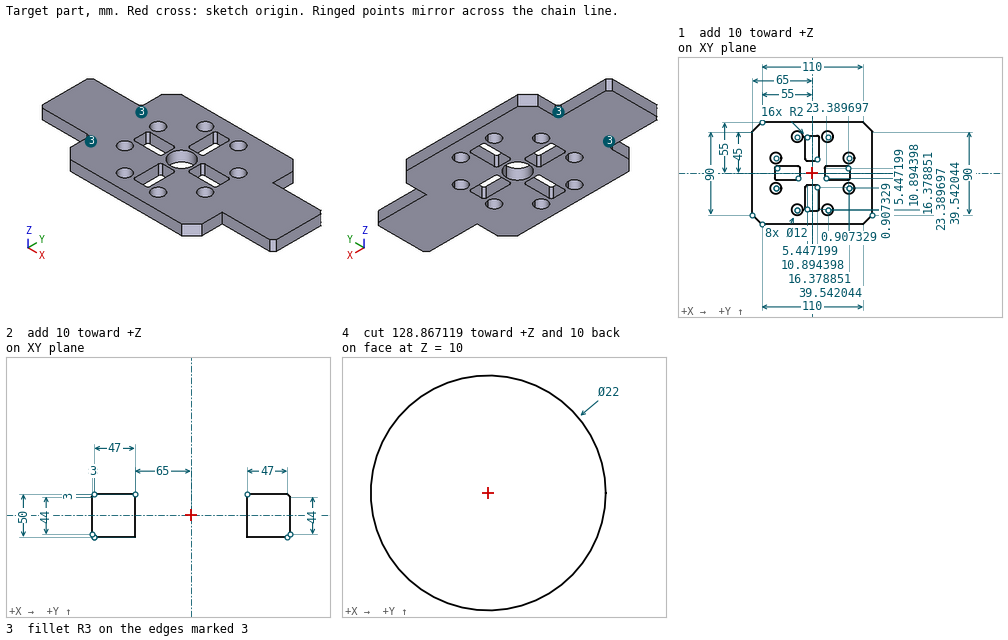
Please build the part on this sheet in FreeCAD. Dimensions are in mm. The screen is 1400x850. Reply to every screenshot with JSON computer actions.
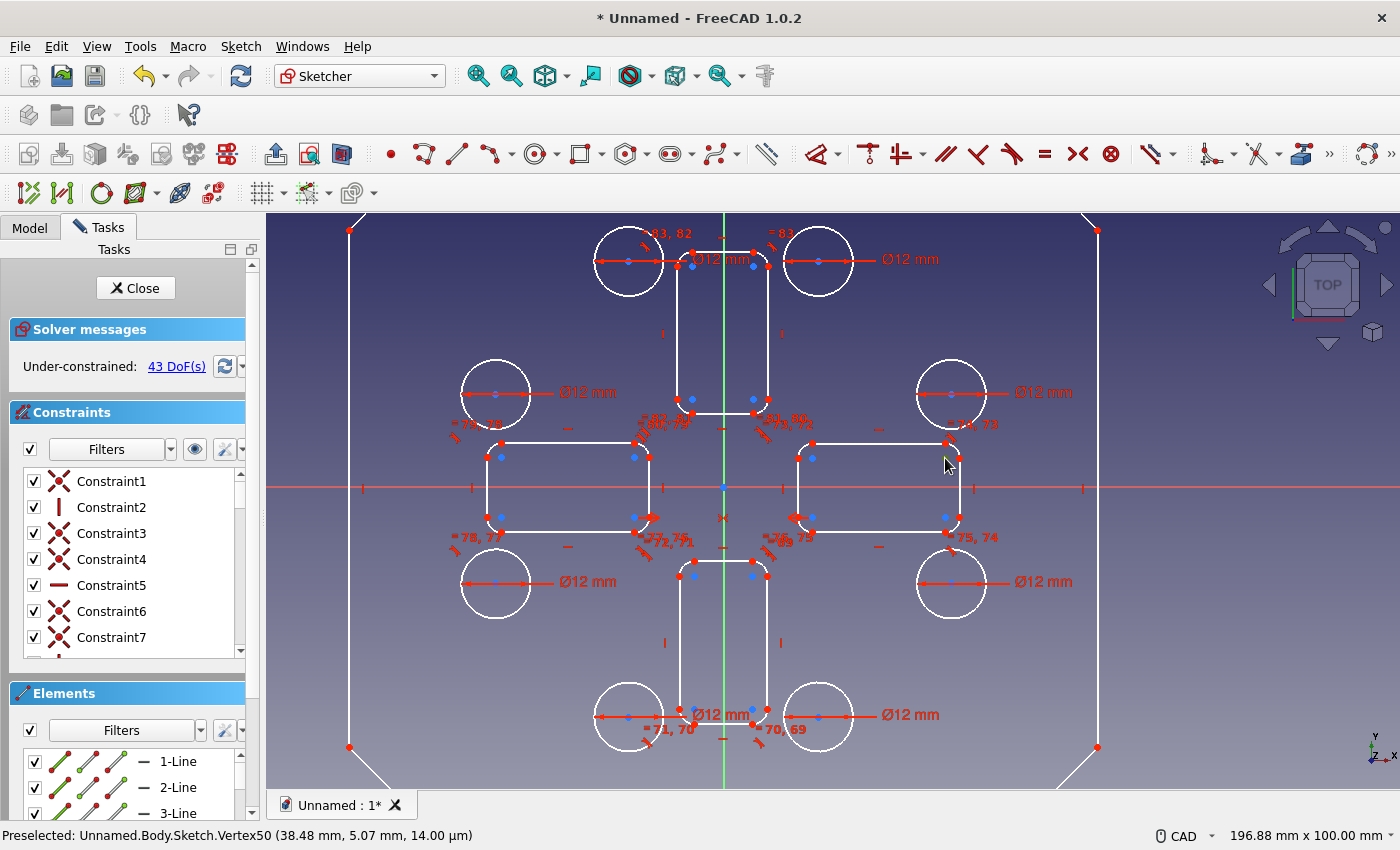
{"action": "left_click", "coordinate": [502, 458]}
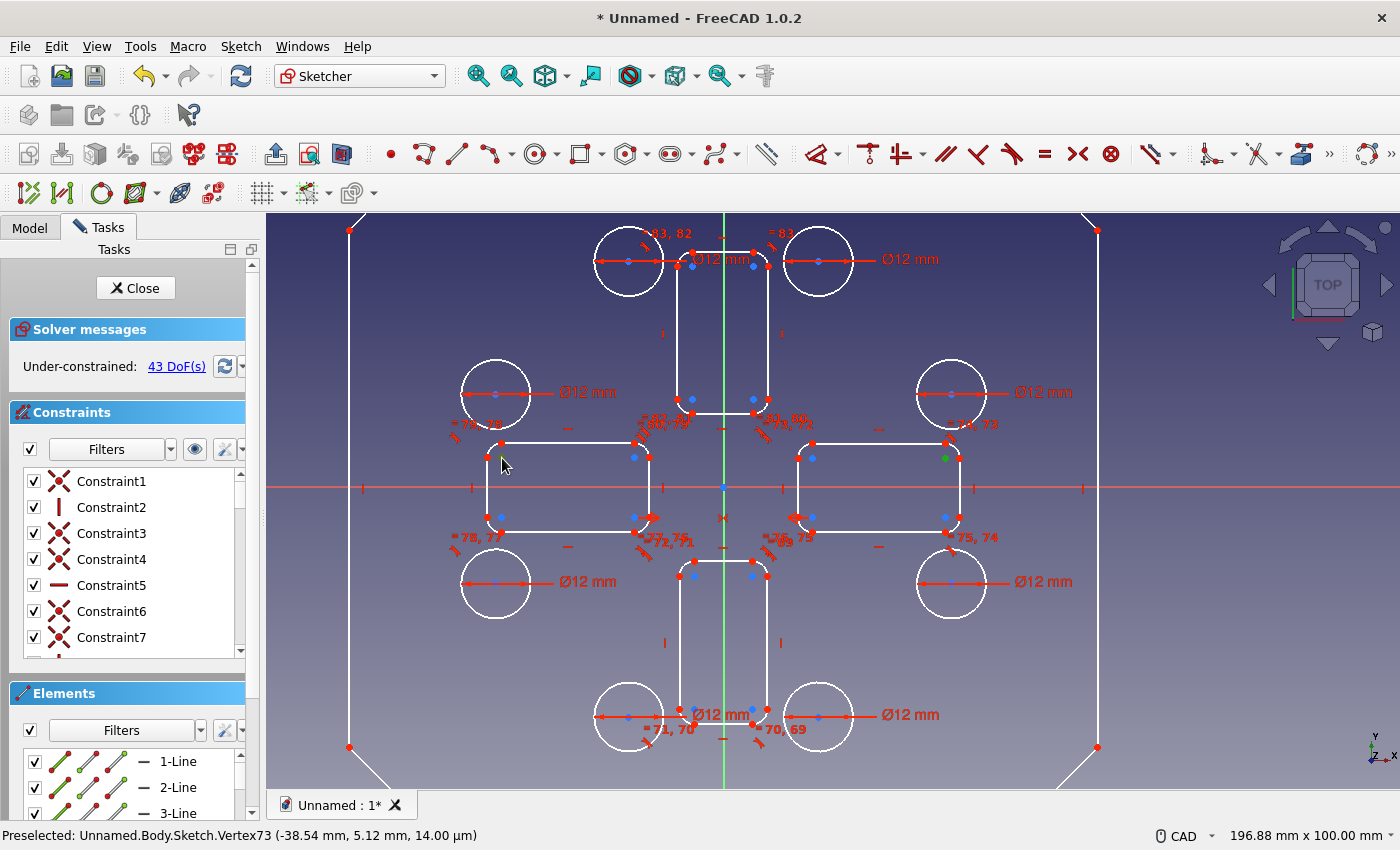
{"action": "left_click", "coordinate": [724, 687]}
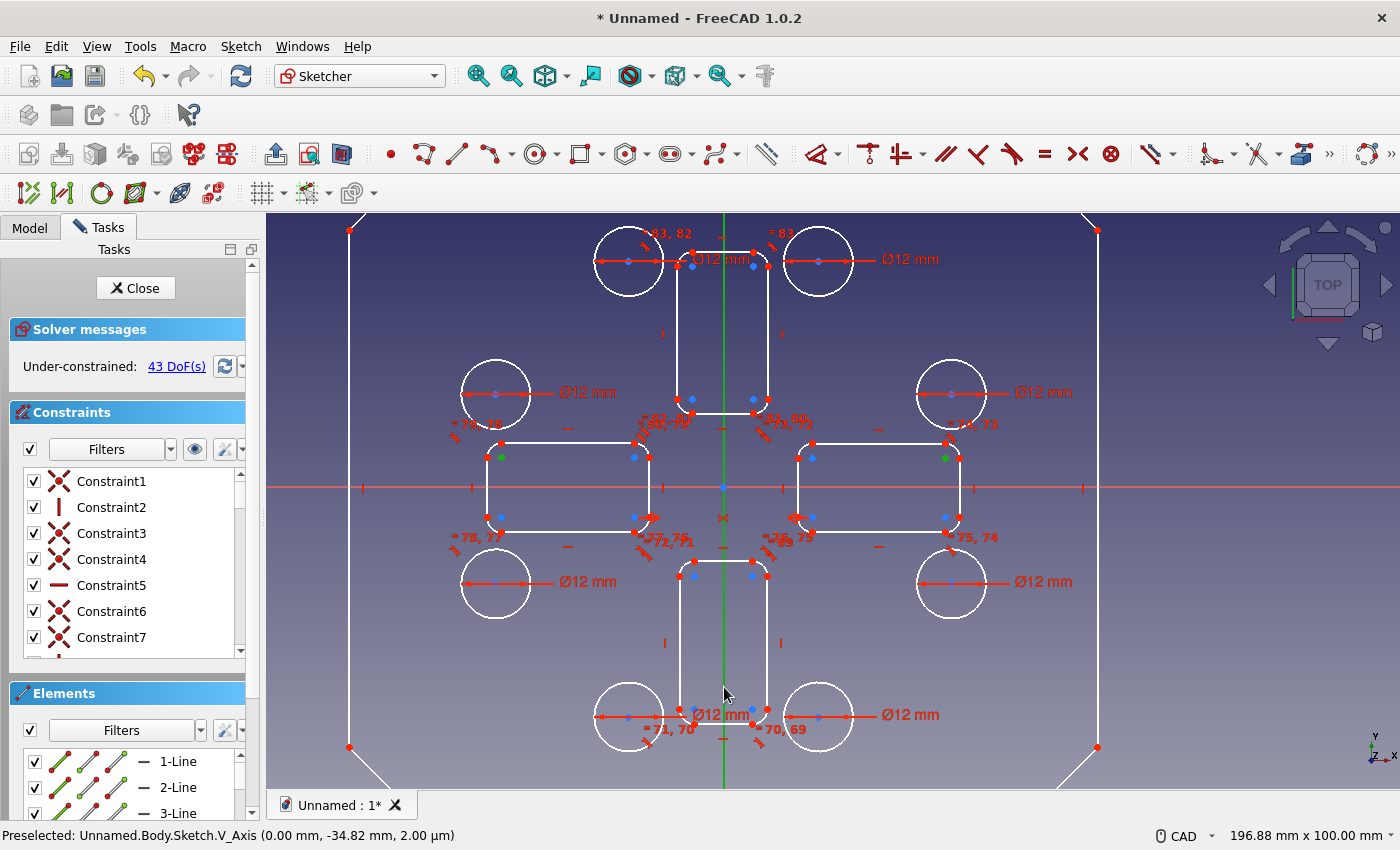
{"action": "left_click", "coordinate": [1078, 154]}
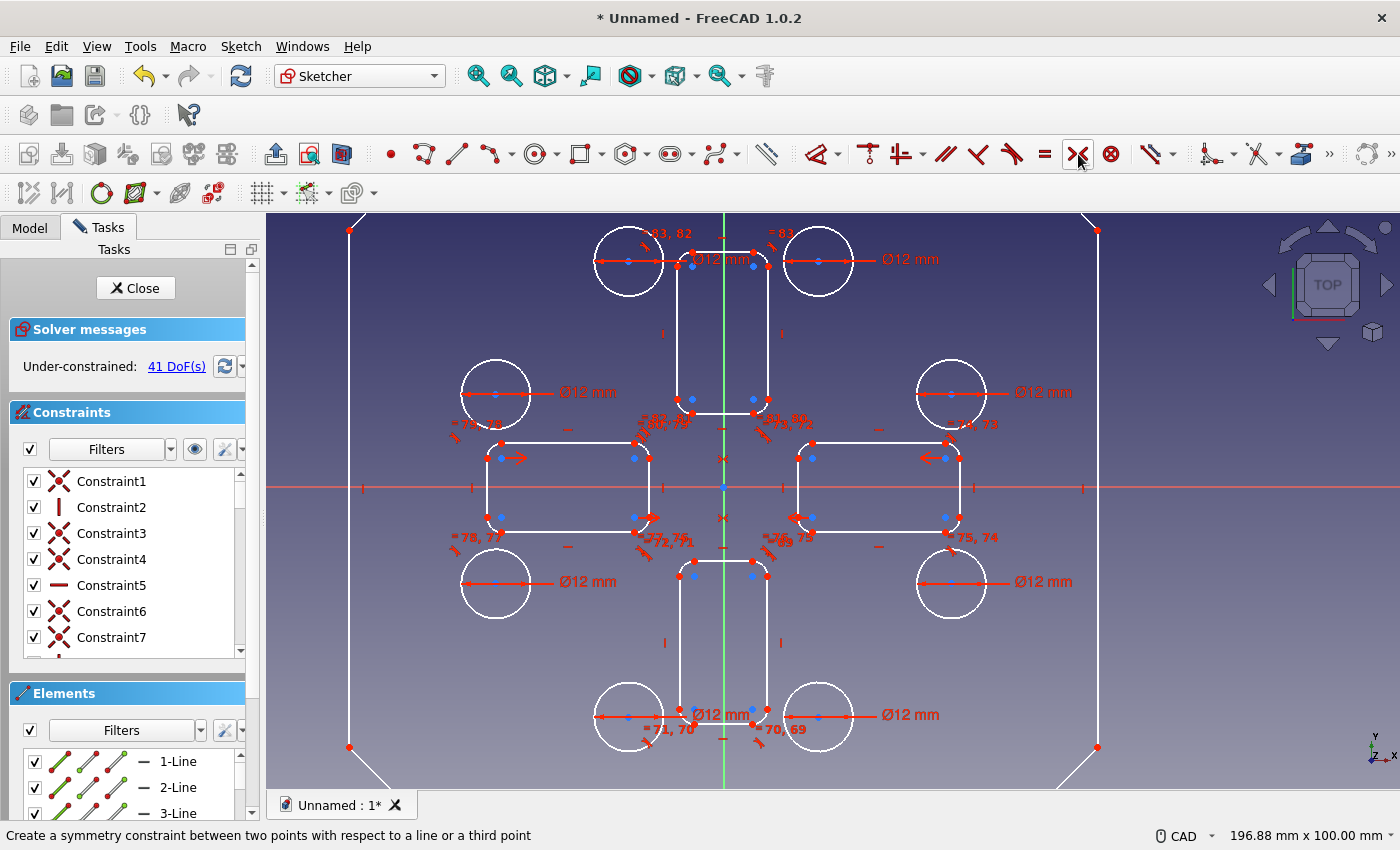
{"action": "left_click", "coordinate": [753, 576]}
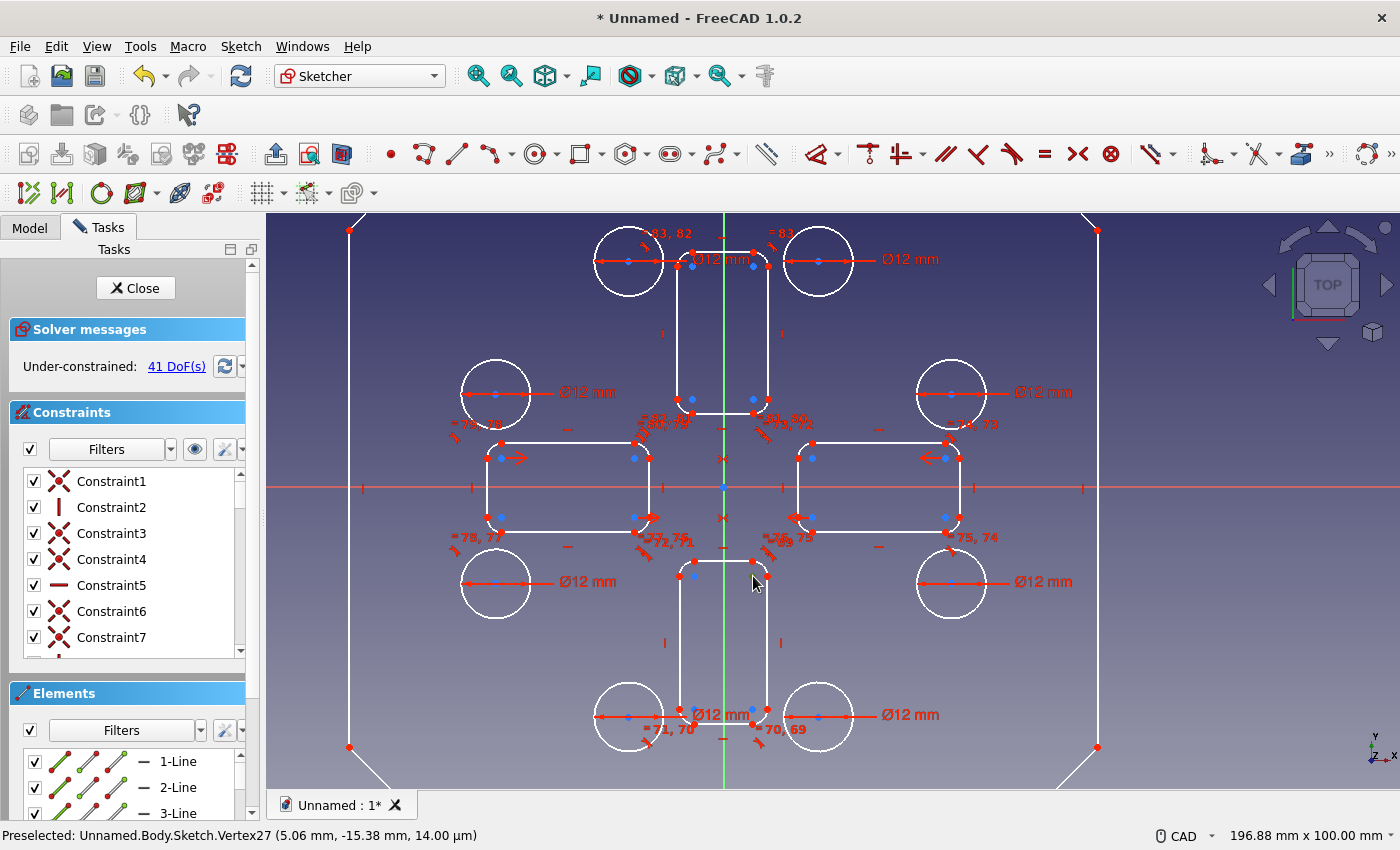
{"action": "left_click", "coordinate": [753, 399]}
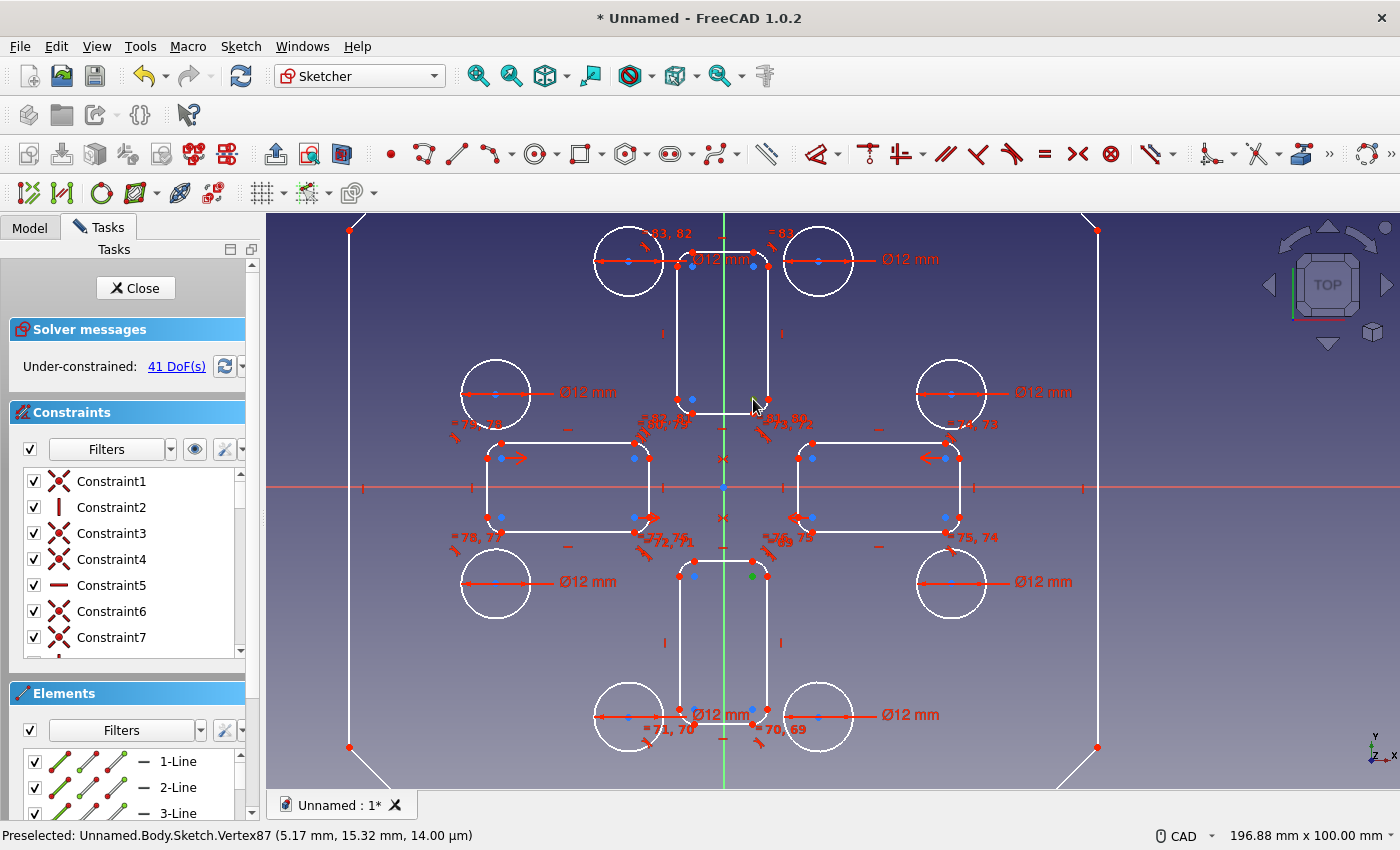
{"action": "left_click", "coordinate": [428, 487]}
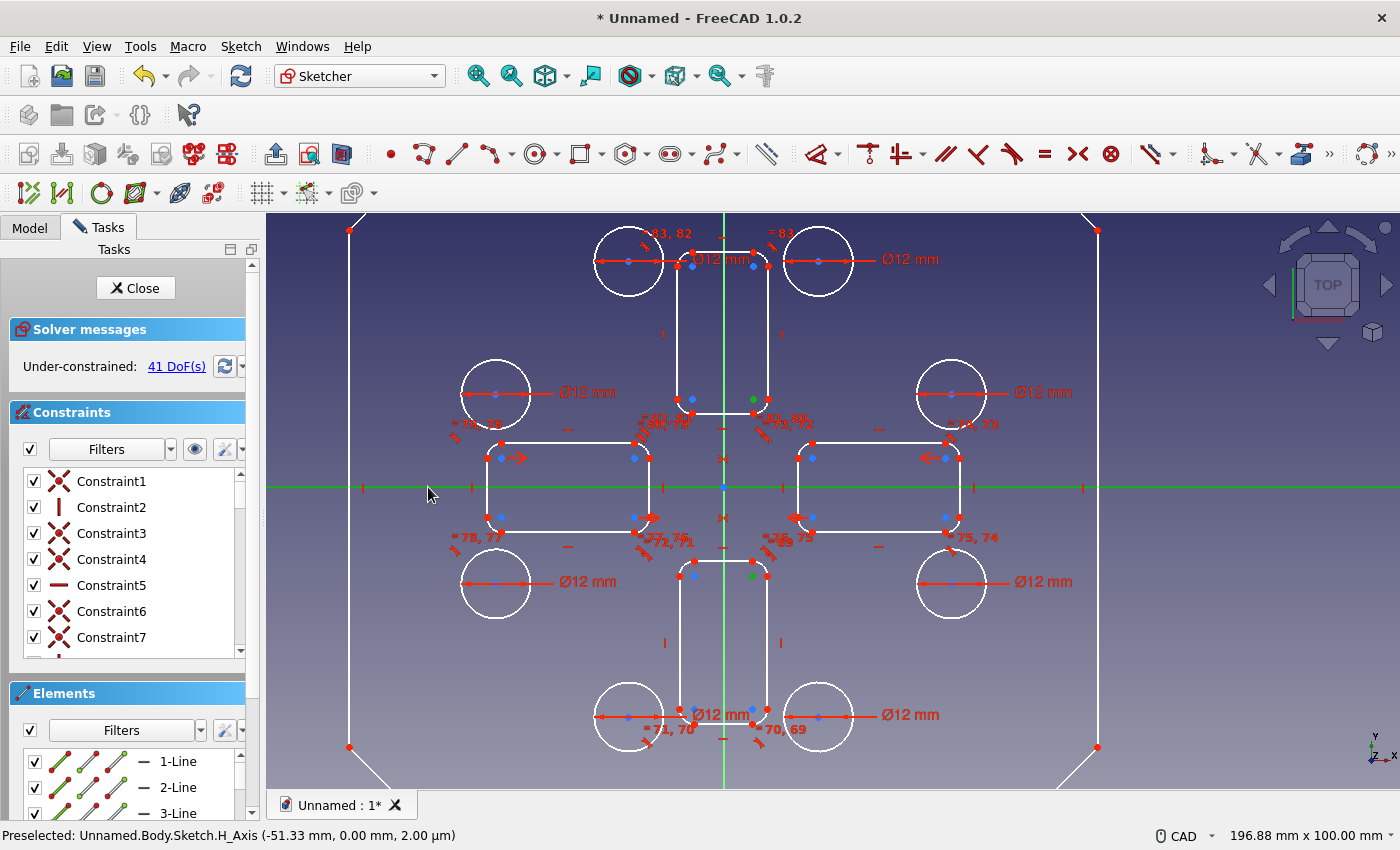
{"action": "left_click", "coordinate": [1078, 154]}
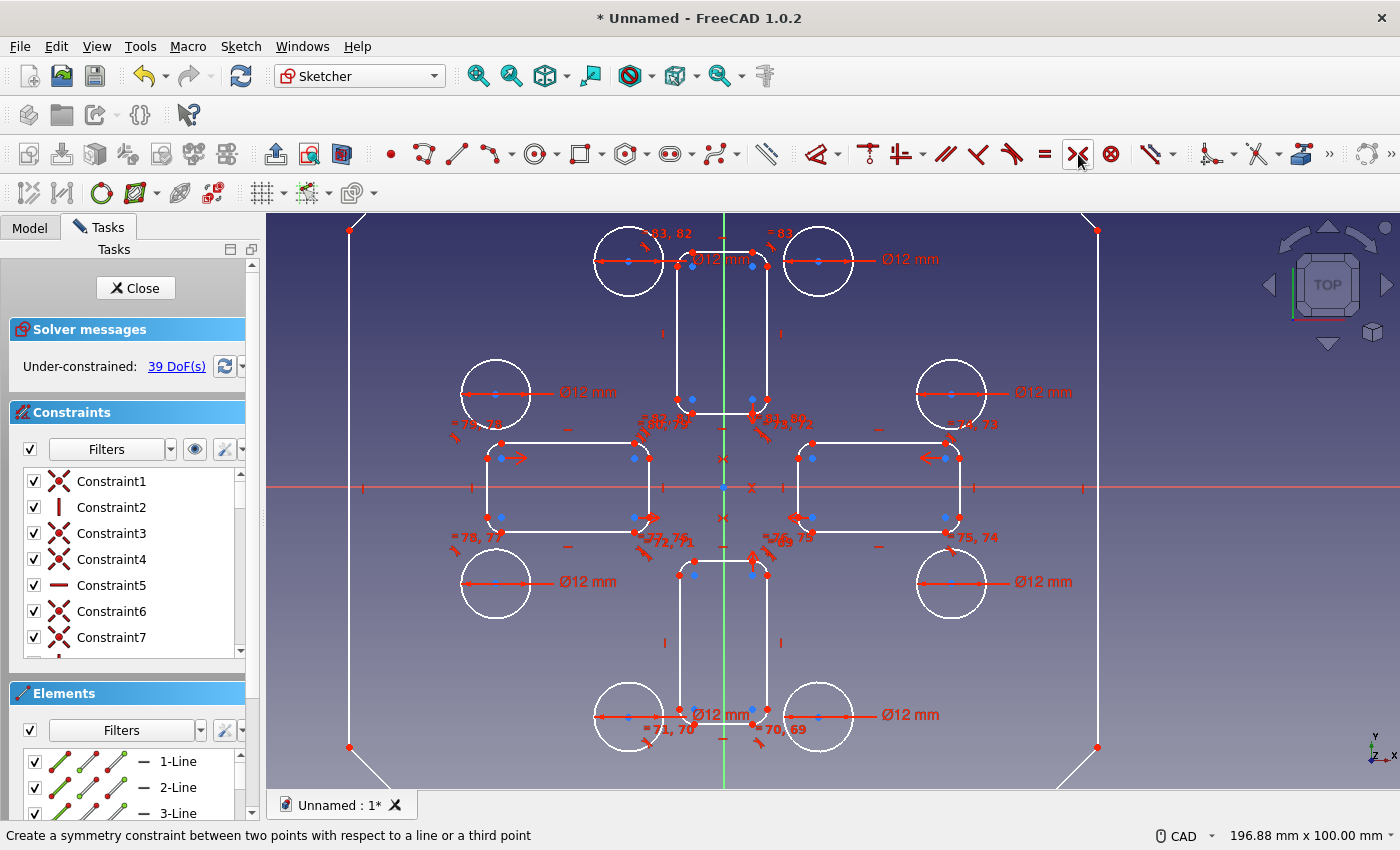
{"action": "left_click", "coordinate": [694, 709]}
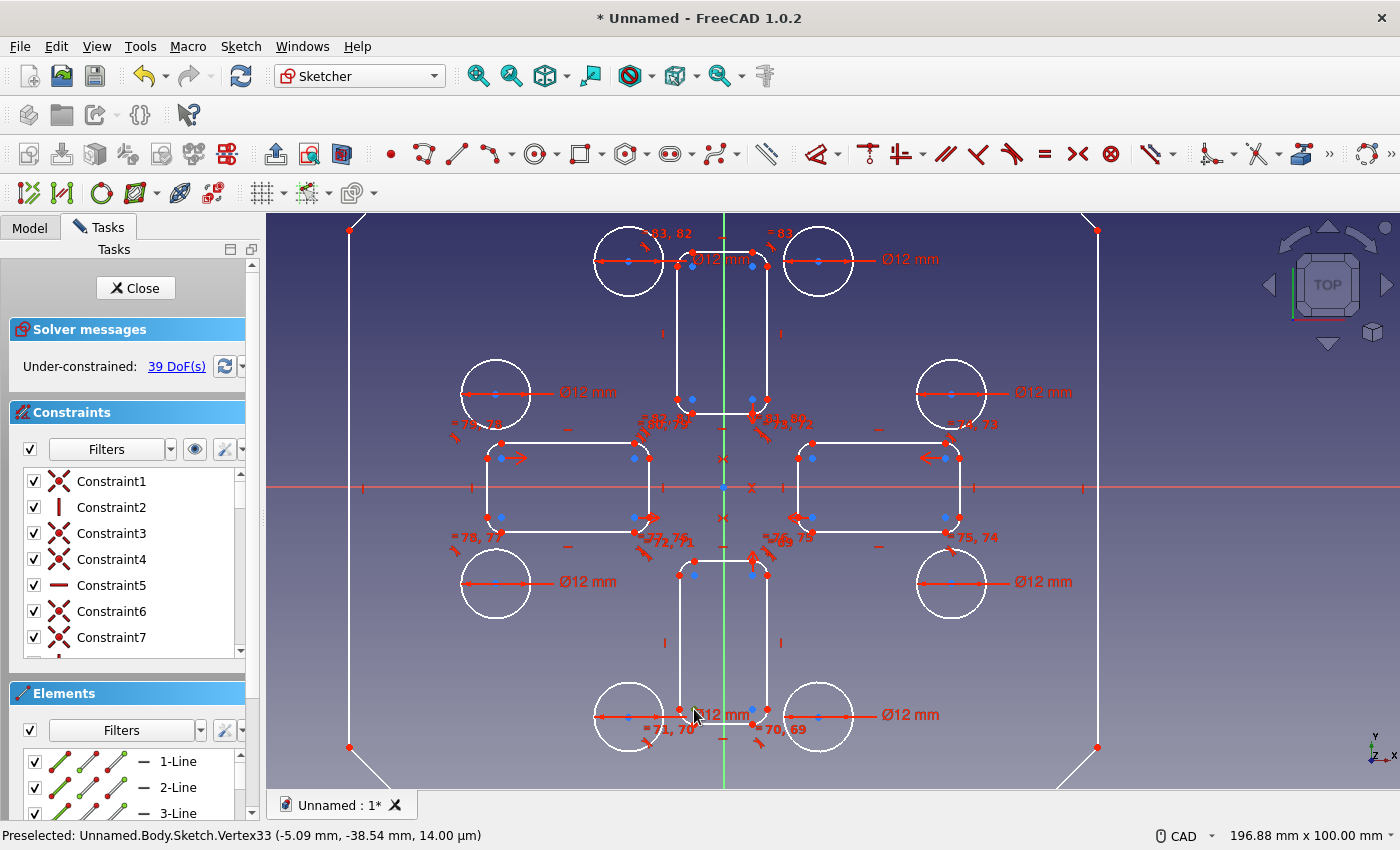
{"action": "left_click", "coordinate": [692, 267]}